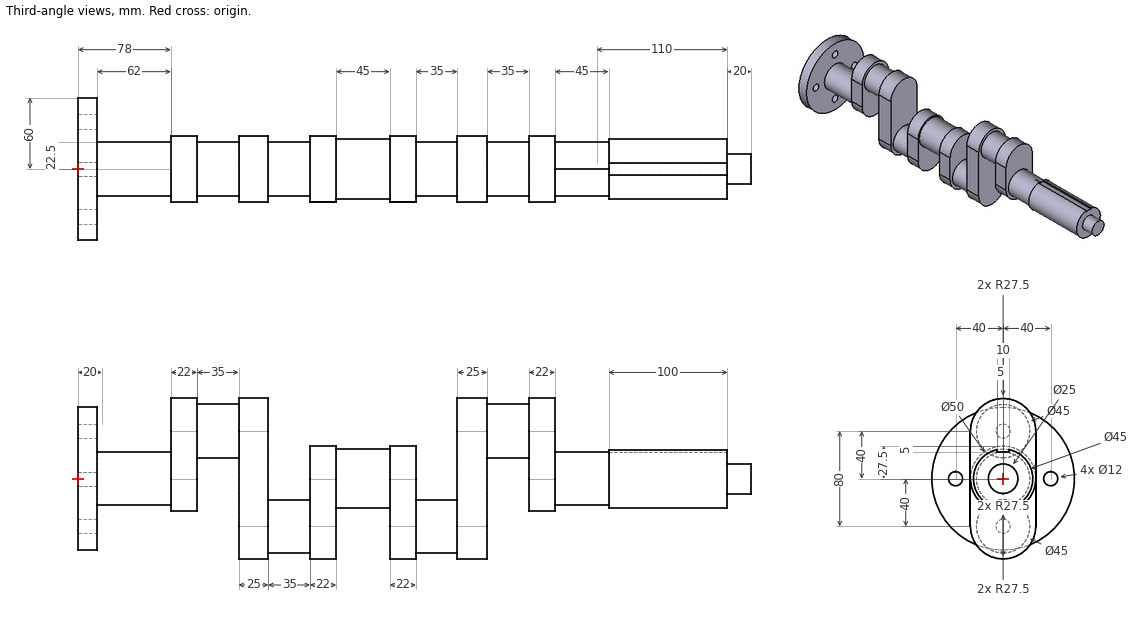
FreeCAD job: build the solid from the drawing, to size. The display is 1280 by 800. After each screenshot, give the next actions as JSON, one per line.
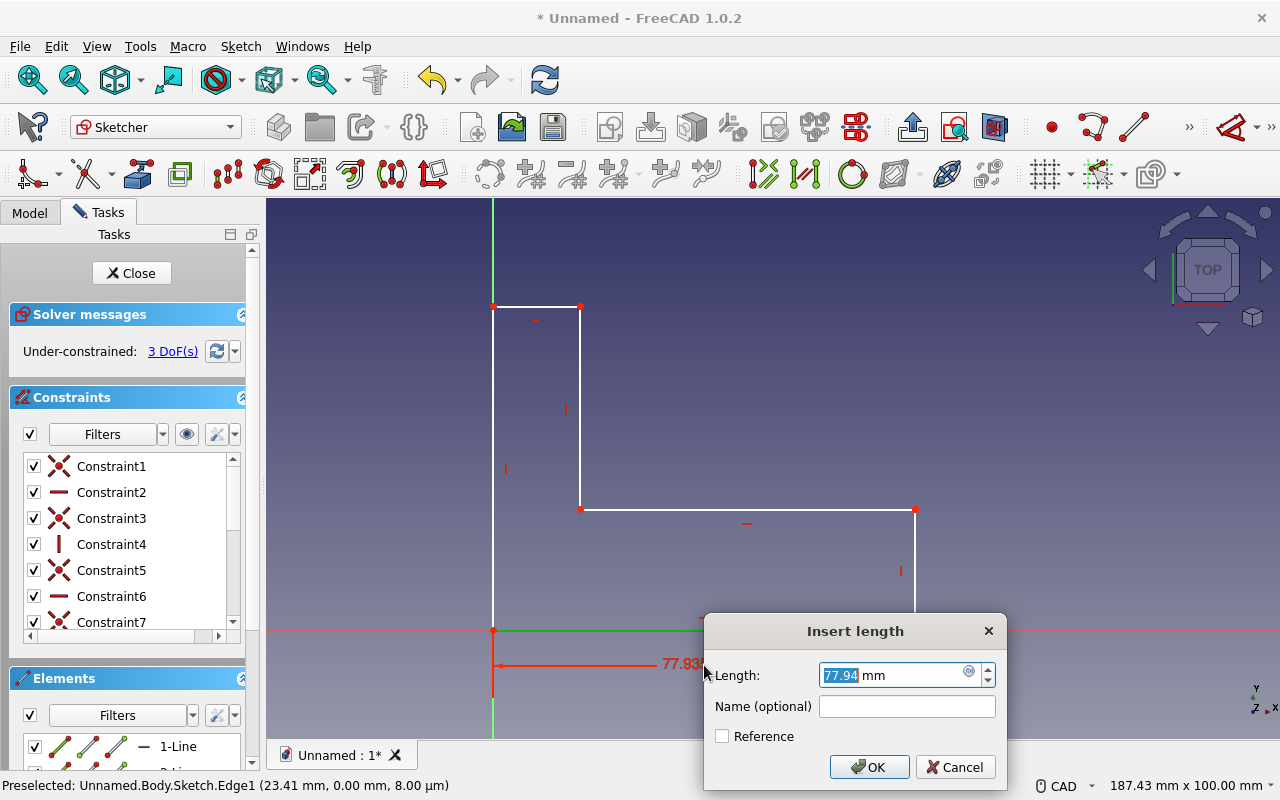
{"action": "type", "text": "78"}
{"action": "key", "text": "Return"}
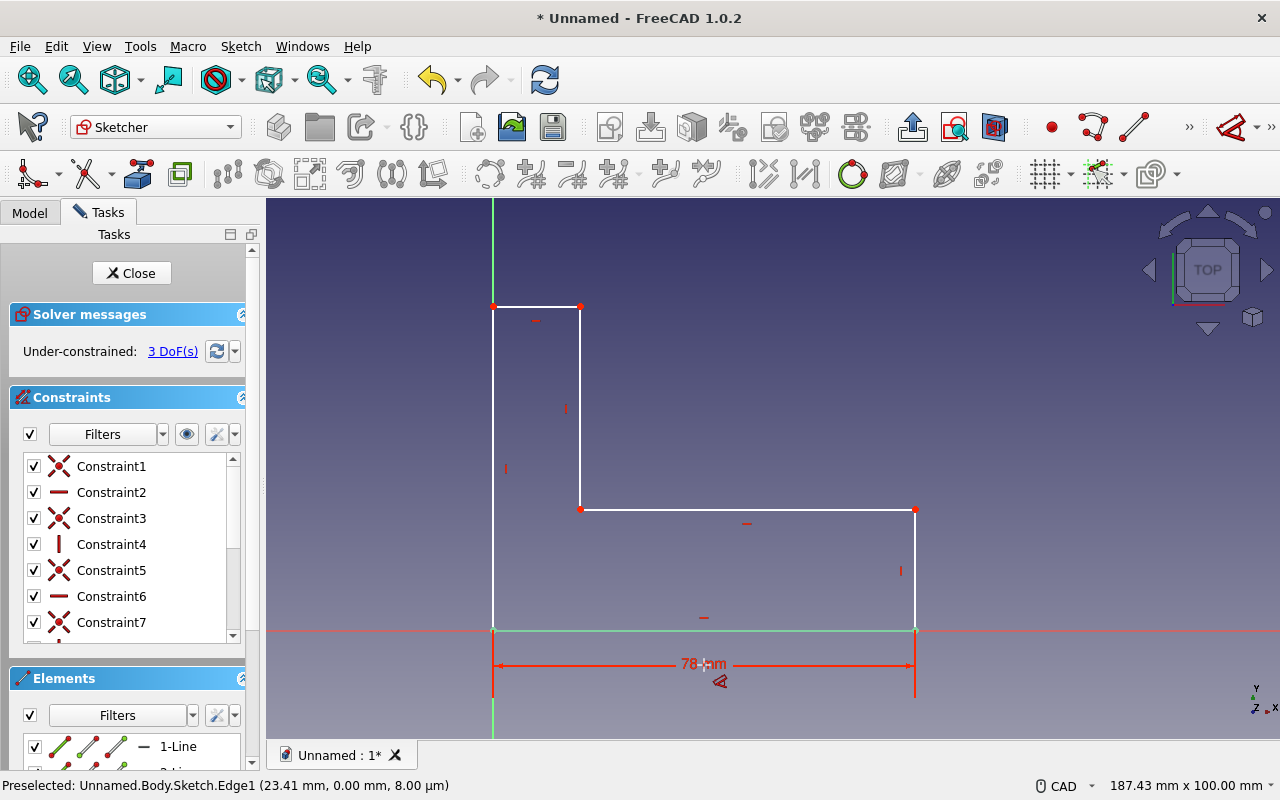
{"action": "left_click", "coordinate": [815, 510]}
{"action": "left_click", "coordinate": [748, 544]}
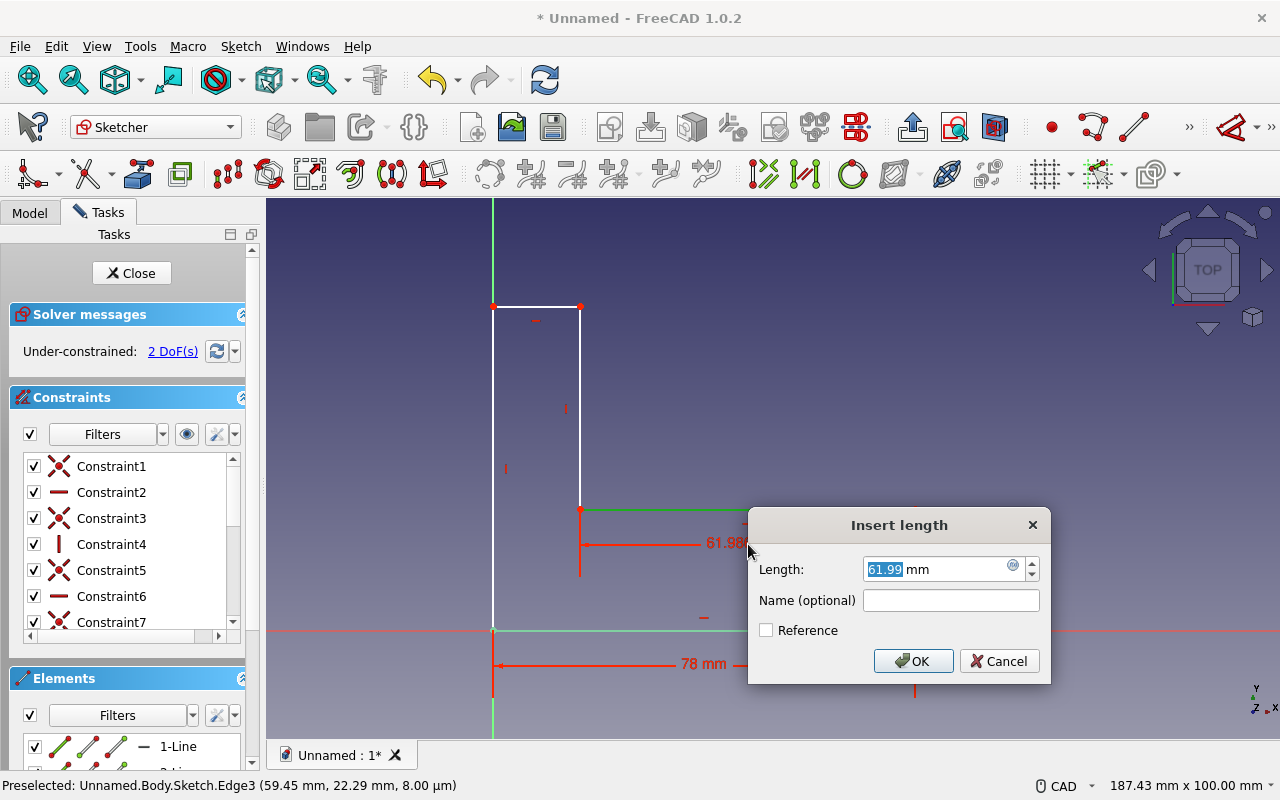
{"action": "type", "text": "62"}
{"action": "key", "text": "Return"}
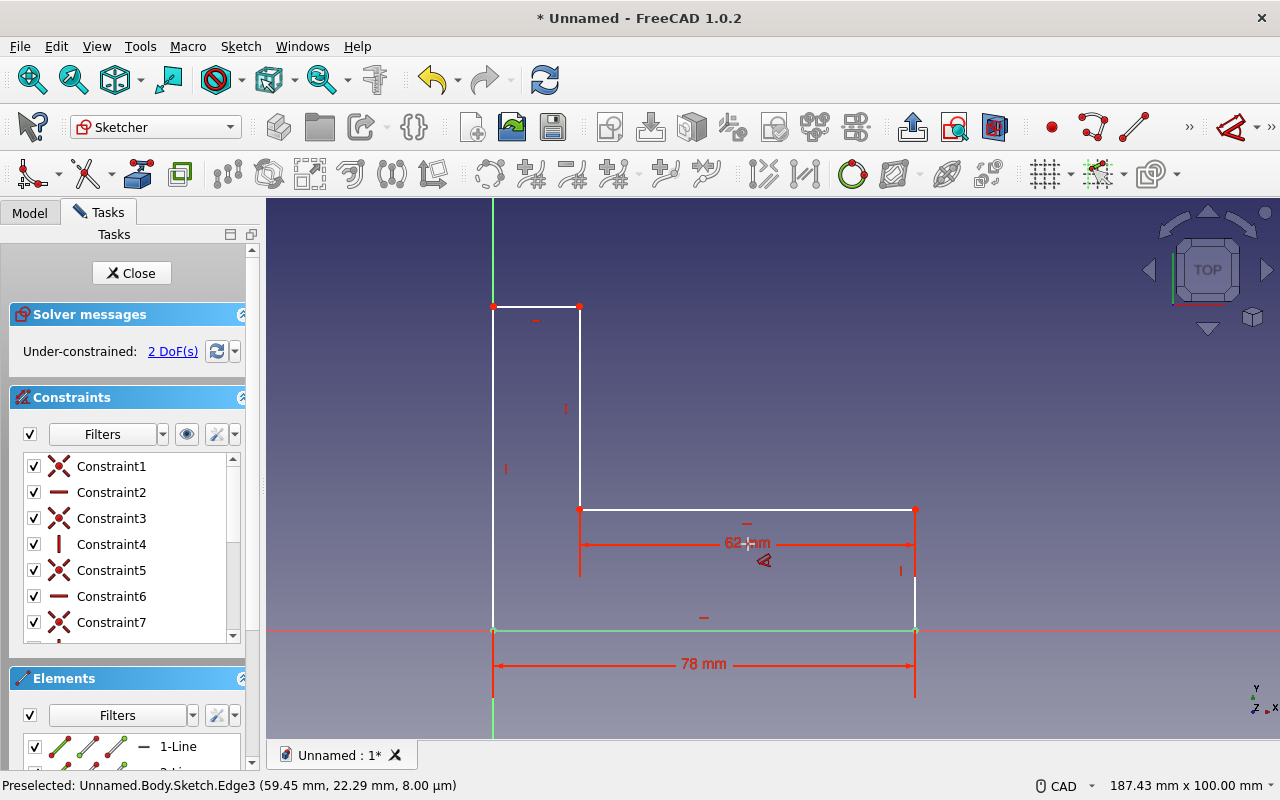
{"action": "left_click", "coordinate": [493, 404]}
{"action": "left_click", "coordinate": [459, 469]}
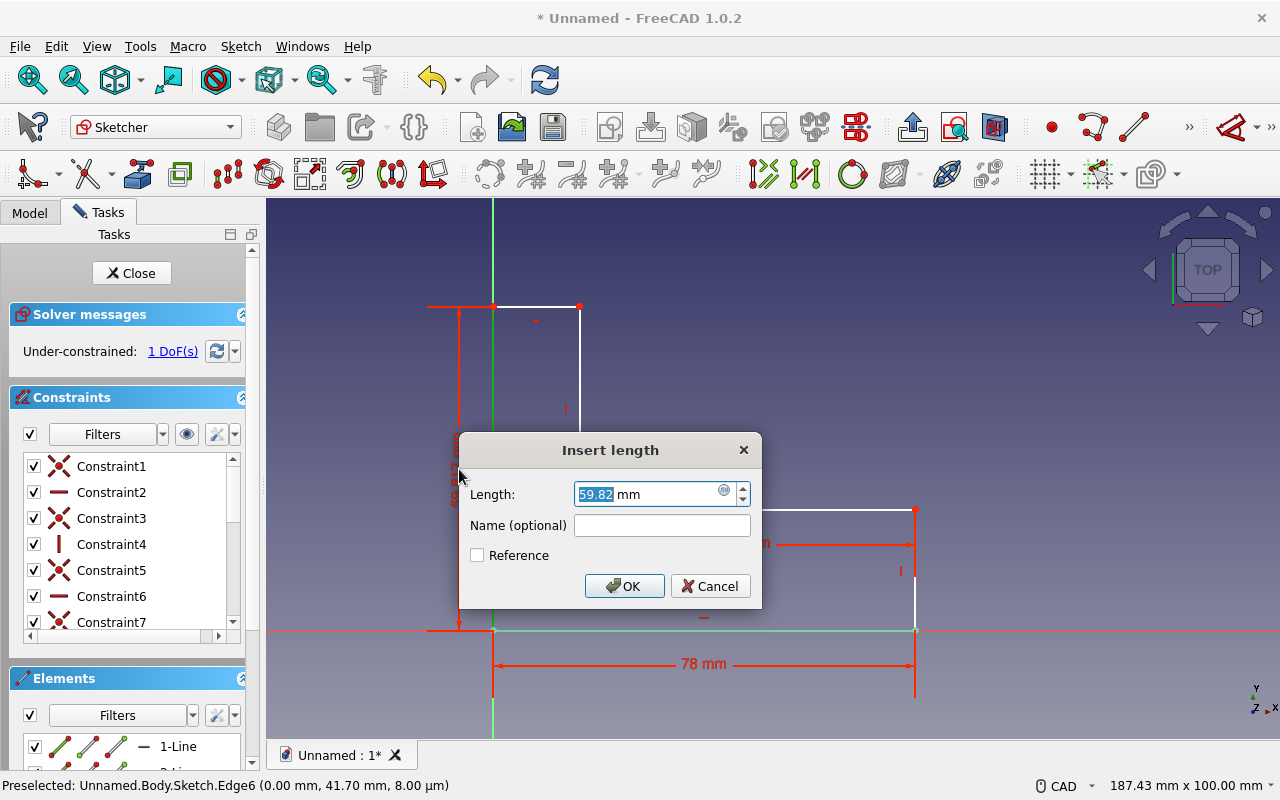
{"action": "type", "text": "60"}
{"action": "key", "text": "Return"}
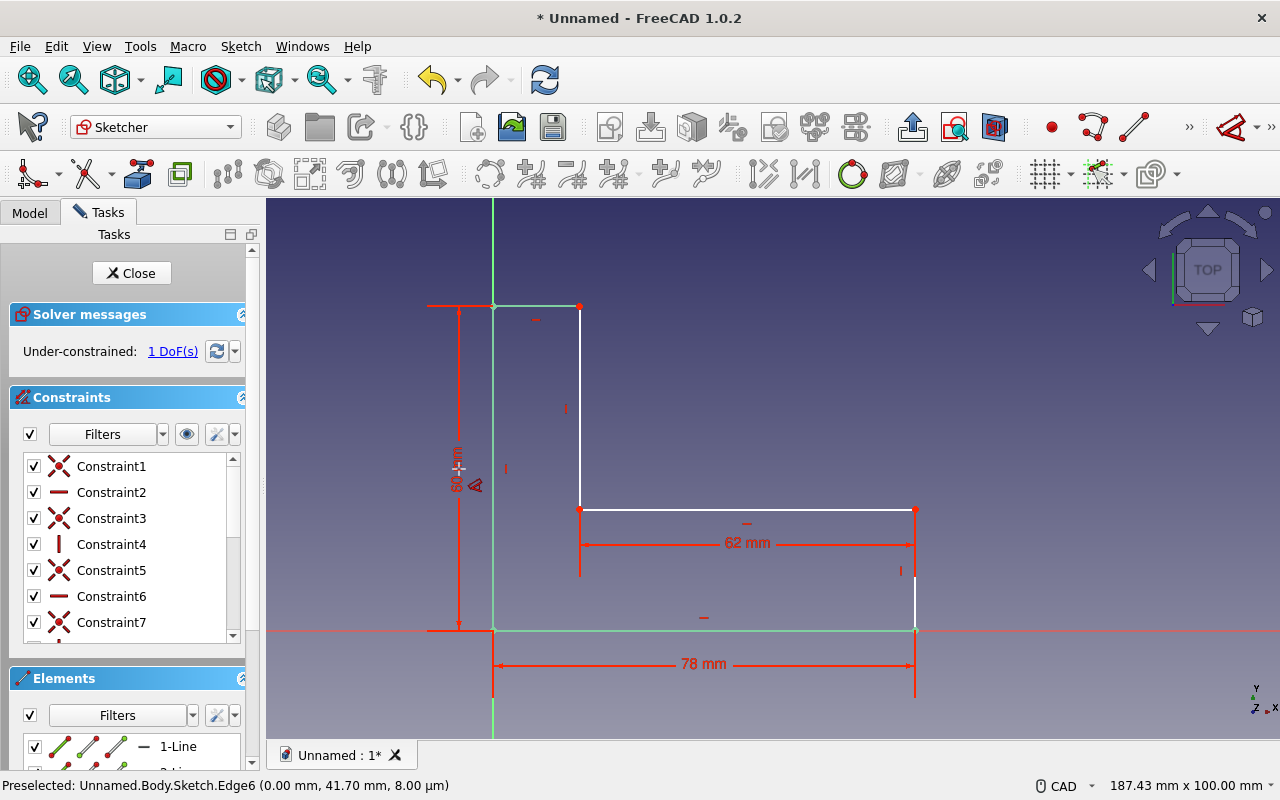
{"action": "left_click", "coordinate": [915, 594]}
{"action": "left_click", "coordinate": [949, 570]}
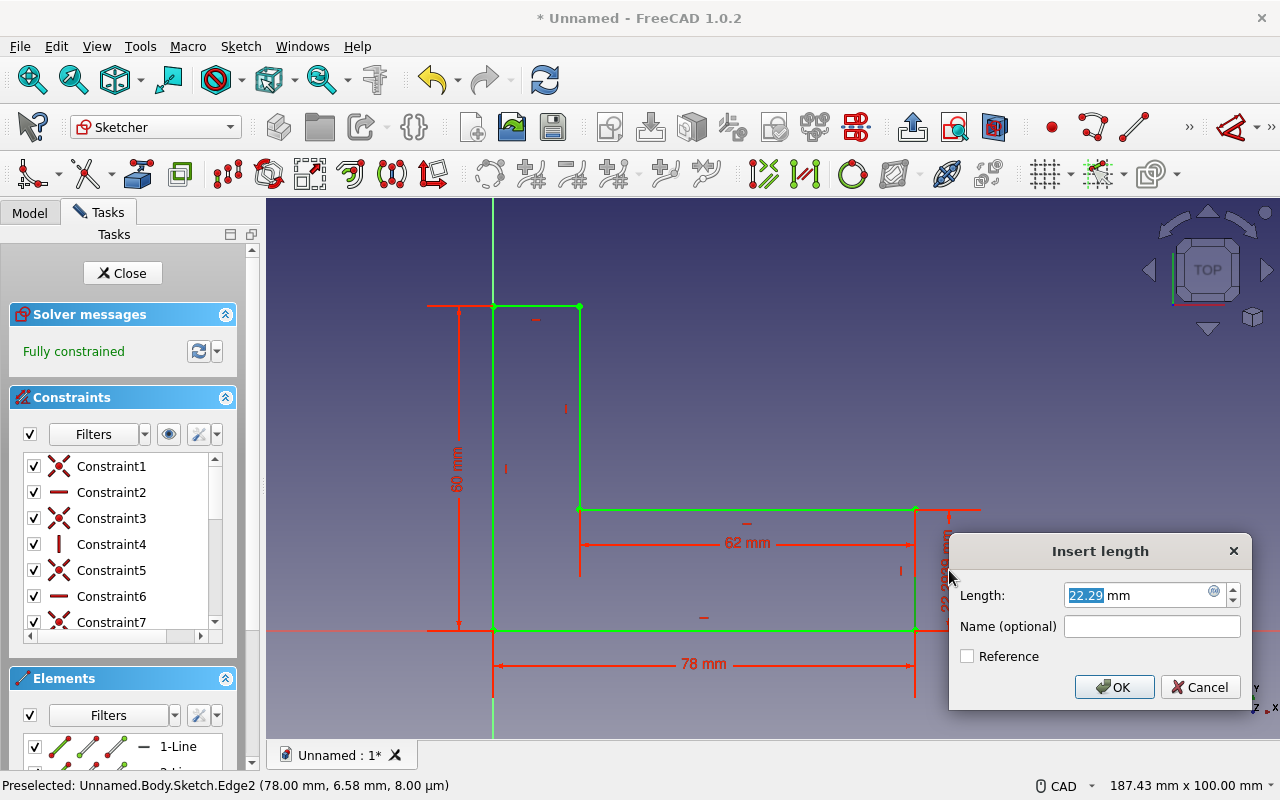
{"action": "type", "text": "22.5"}
{"action": "key", "text": "Return"}
{"action": "key", "text": "Escape"}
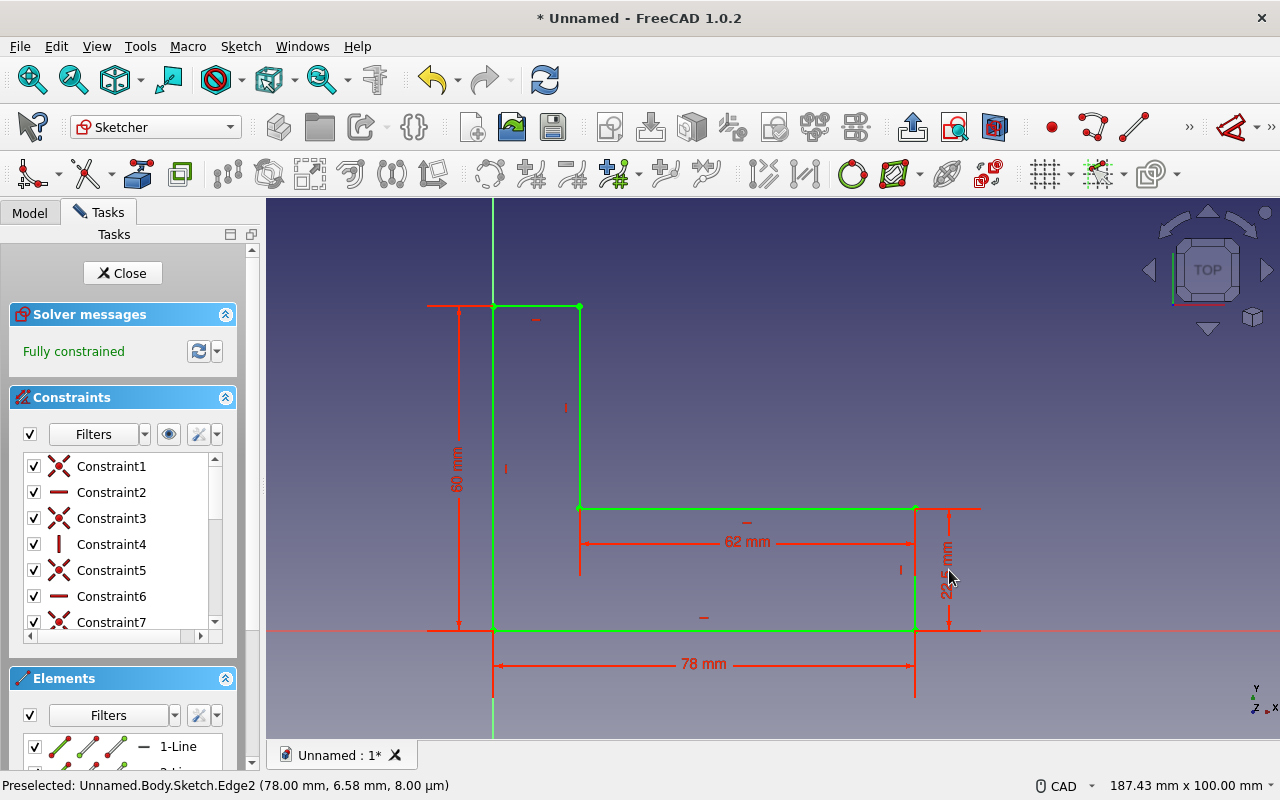
{"action": "left_click", "coordinate": [123, 273]}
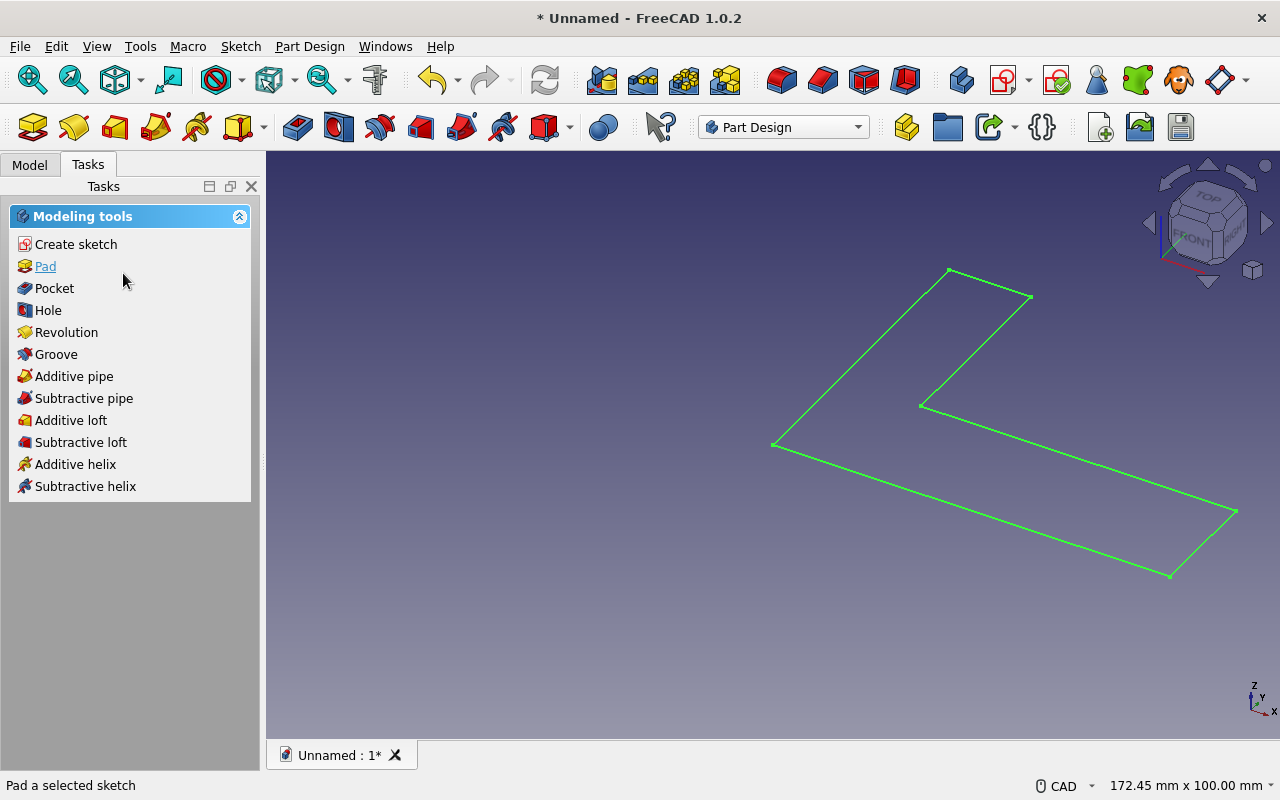
{"action": "left_click", "coordinate": [74, 128]}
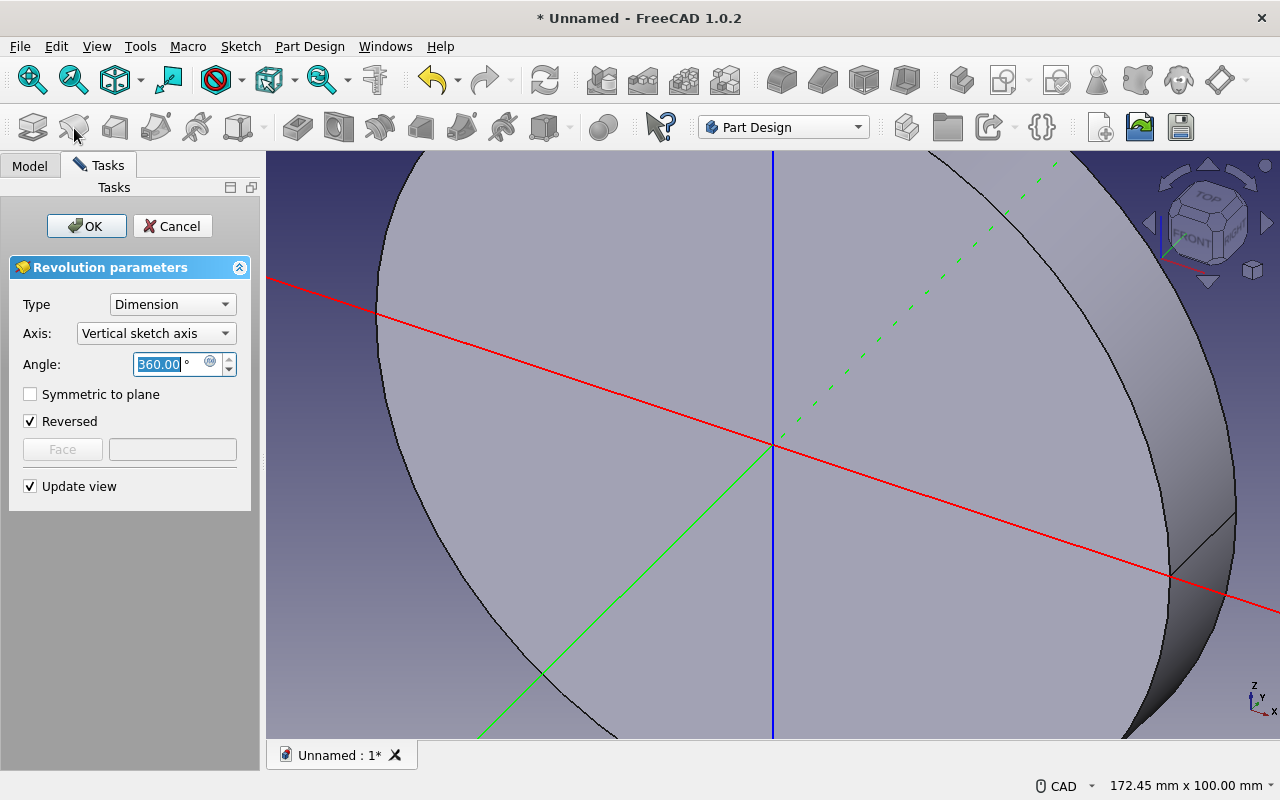
{"action": "left_click", "coordinate": [157, 334]}